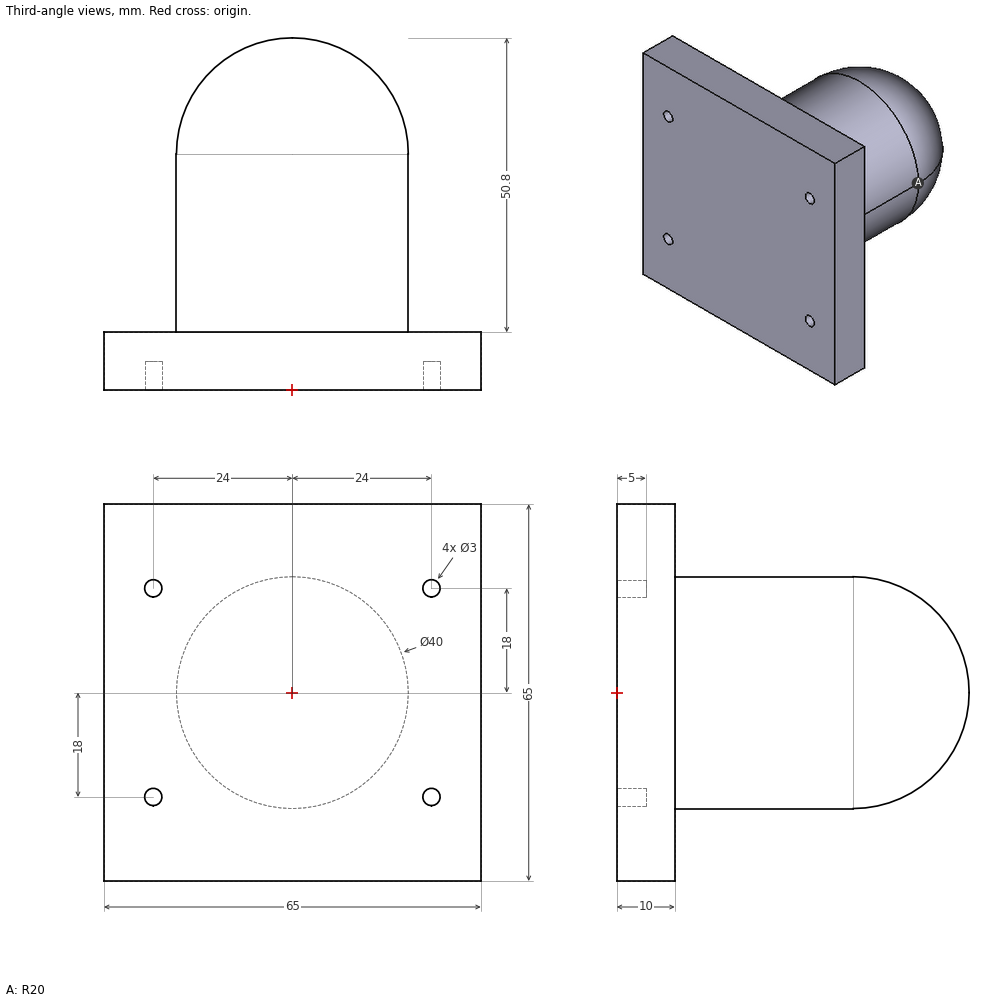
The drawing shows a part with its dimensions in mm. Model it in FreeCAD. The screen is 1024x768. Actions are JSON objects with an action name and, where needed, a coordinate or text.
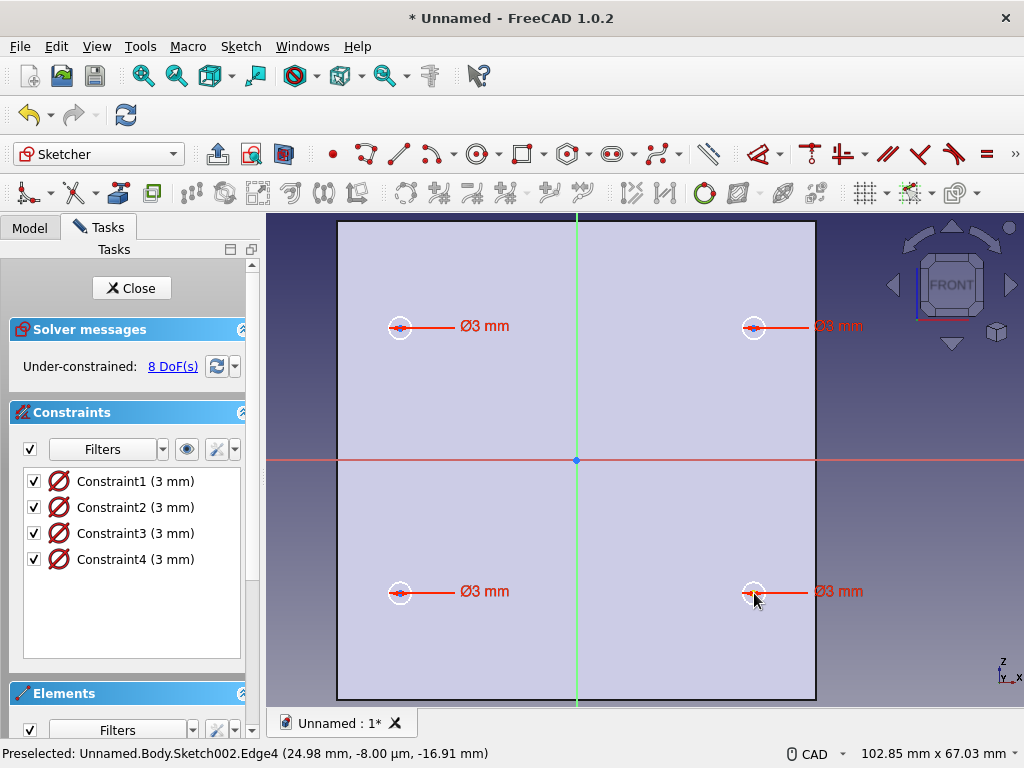
{"action": "left_click", "coordinate": [754, 328]}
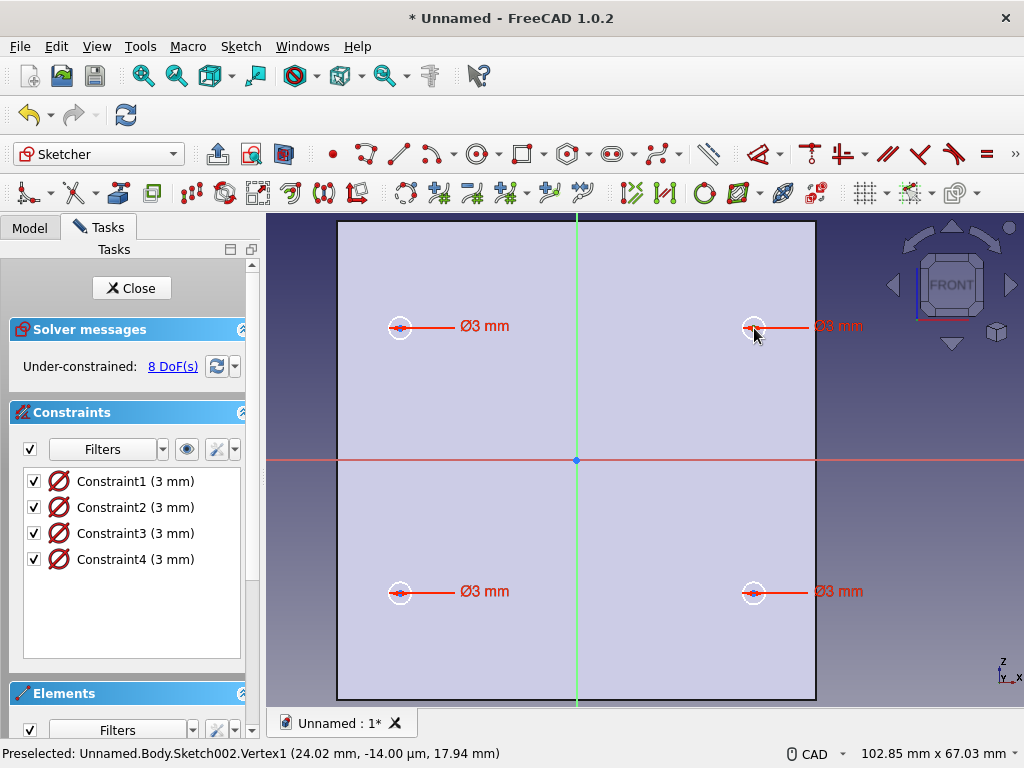
{"action": "left_click", "coordinate": [400, 328]}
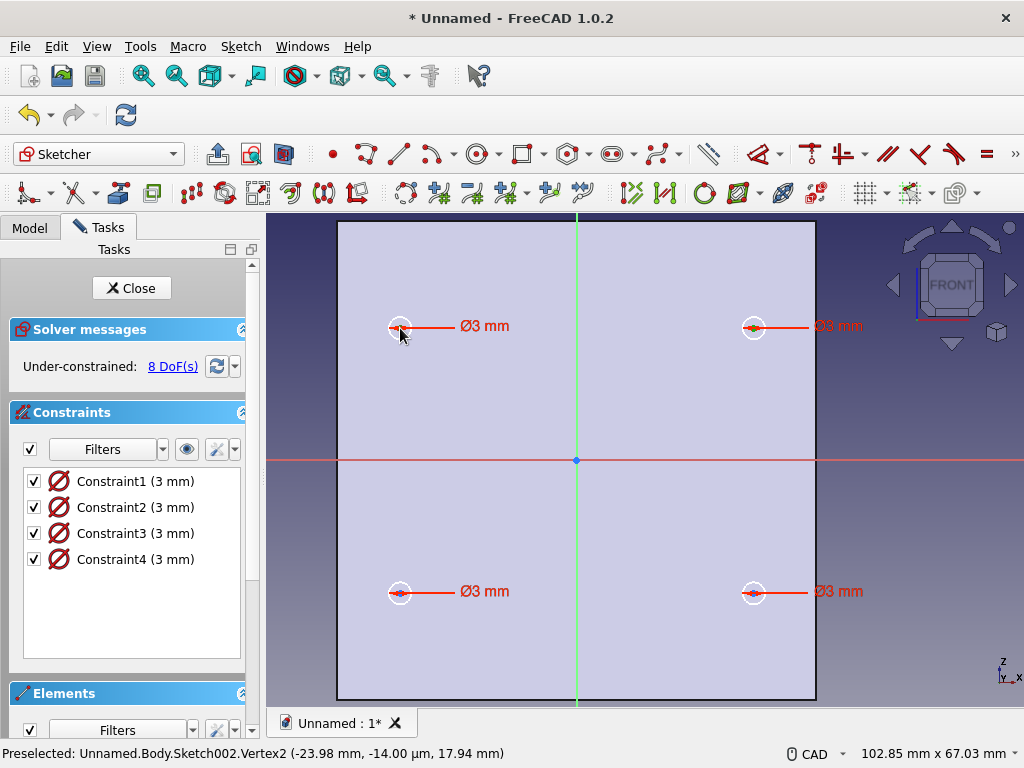
{"action": "key", "text": "h"}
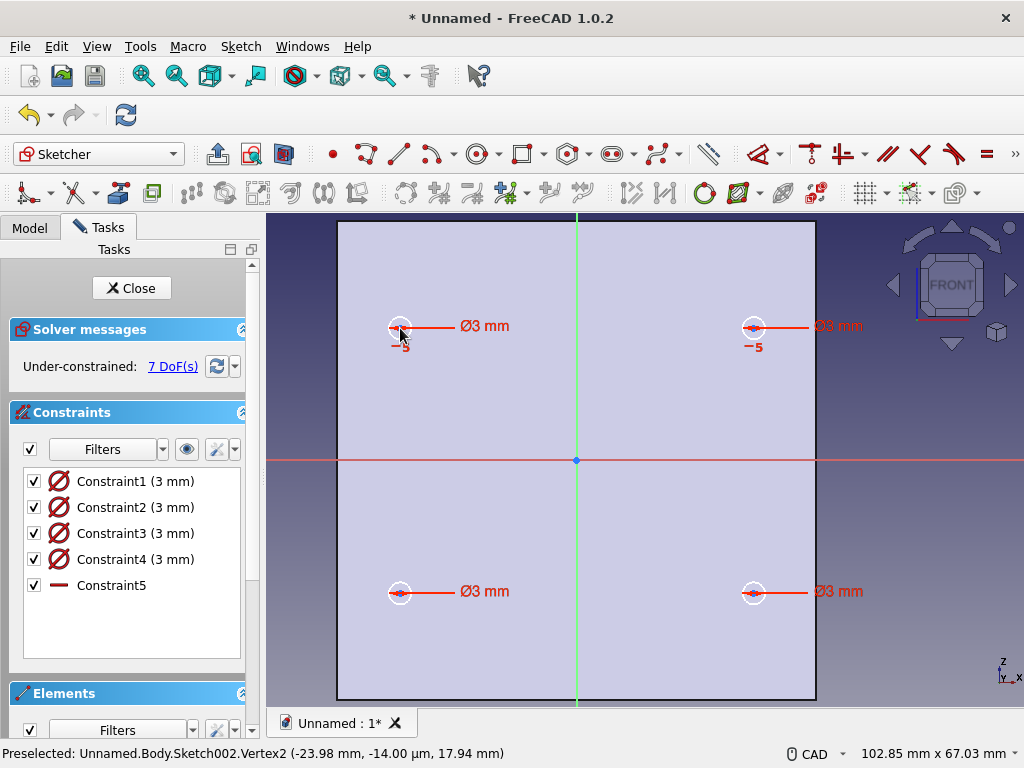
{"action": "left_click", "coordinate": [400, 328]}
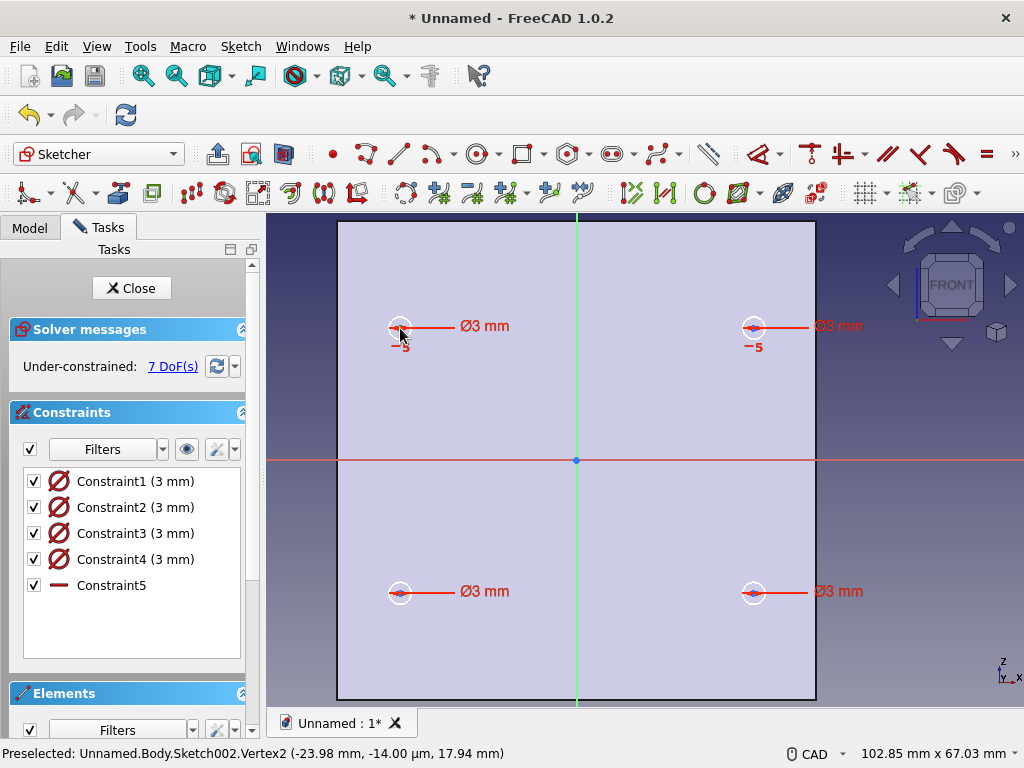
{"action": "left_click", "coordinate": [400, 593]}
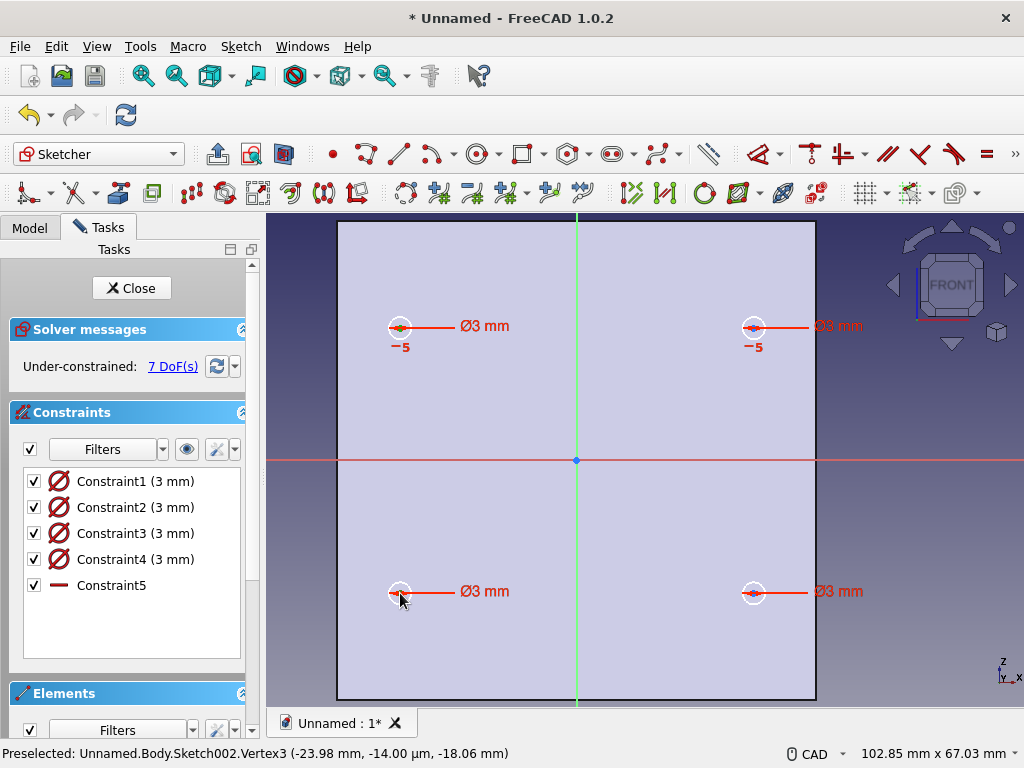
{"action": "left_click", "coordinate": [864, 154]}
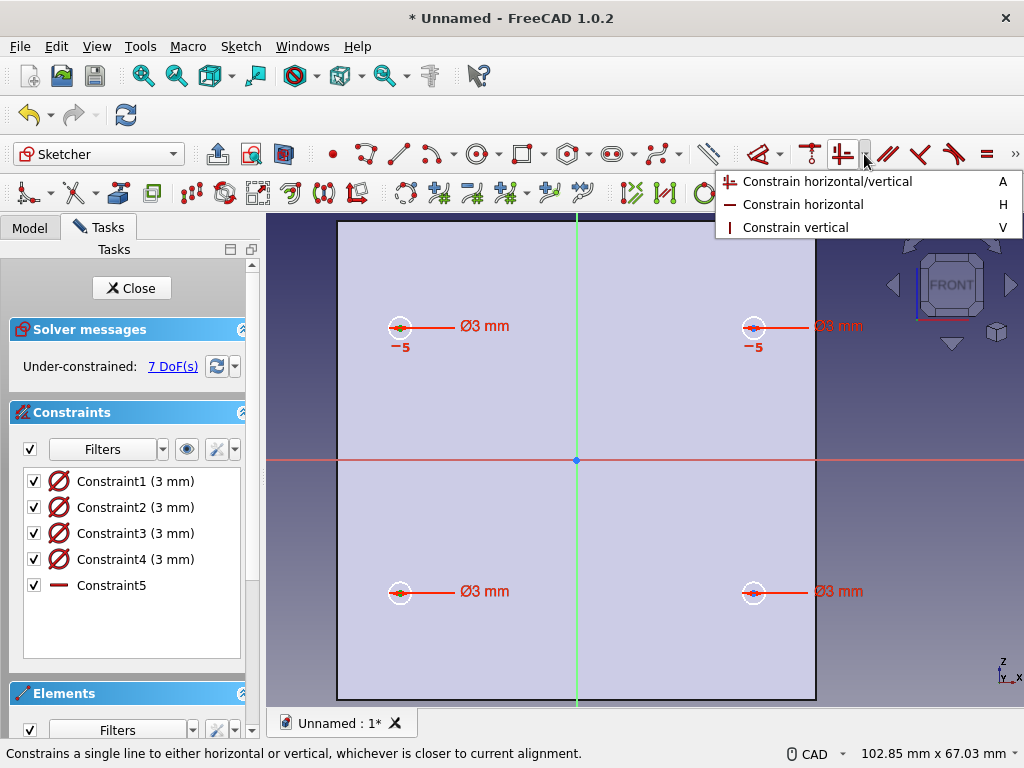
{"action": "left_click", "coordinate": [869, 228]}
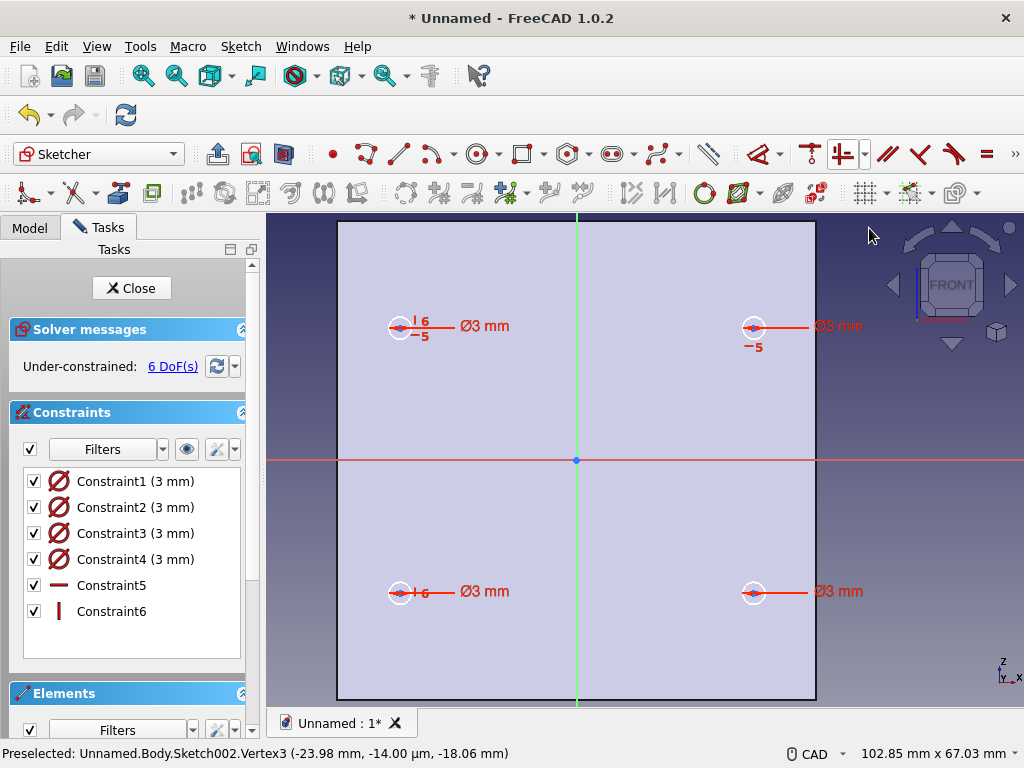
{"action": "left_click", "coordinate": [754, 328]}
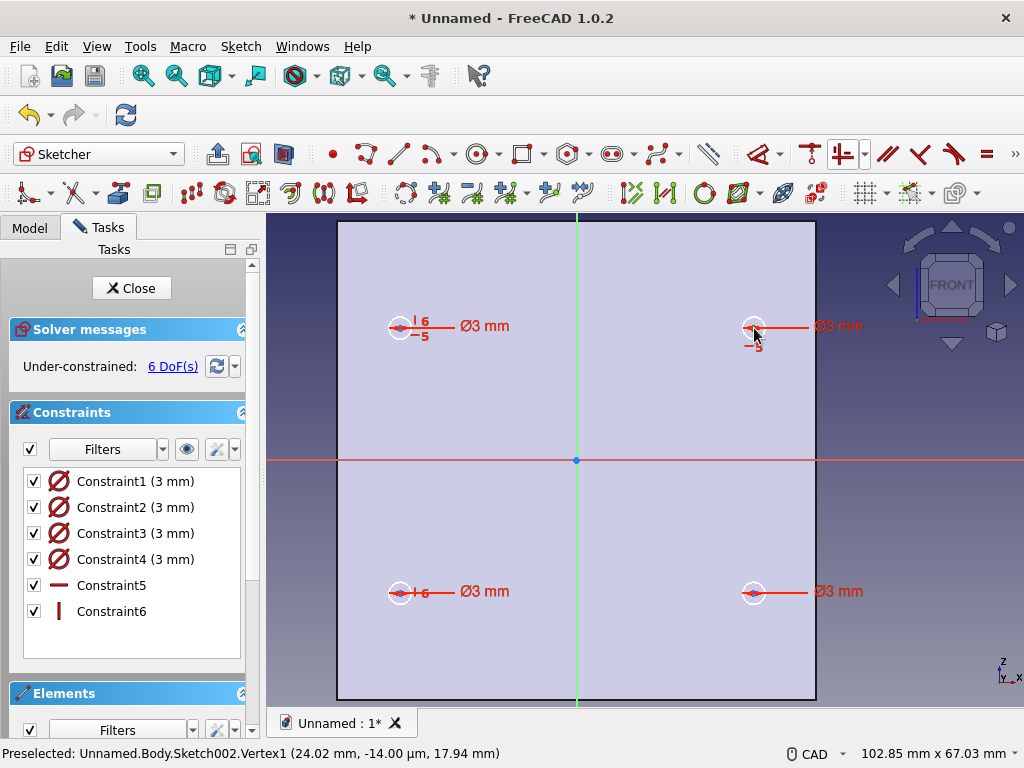
{"action": "left_click", "coordinate": [754, 593]}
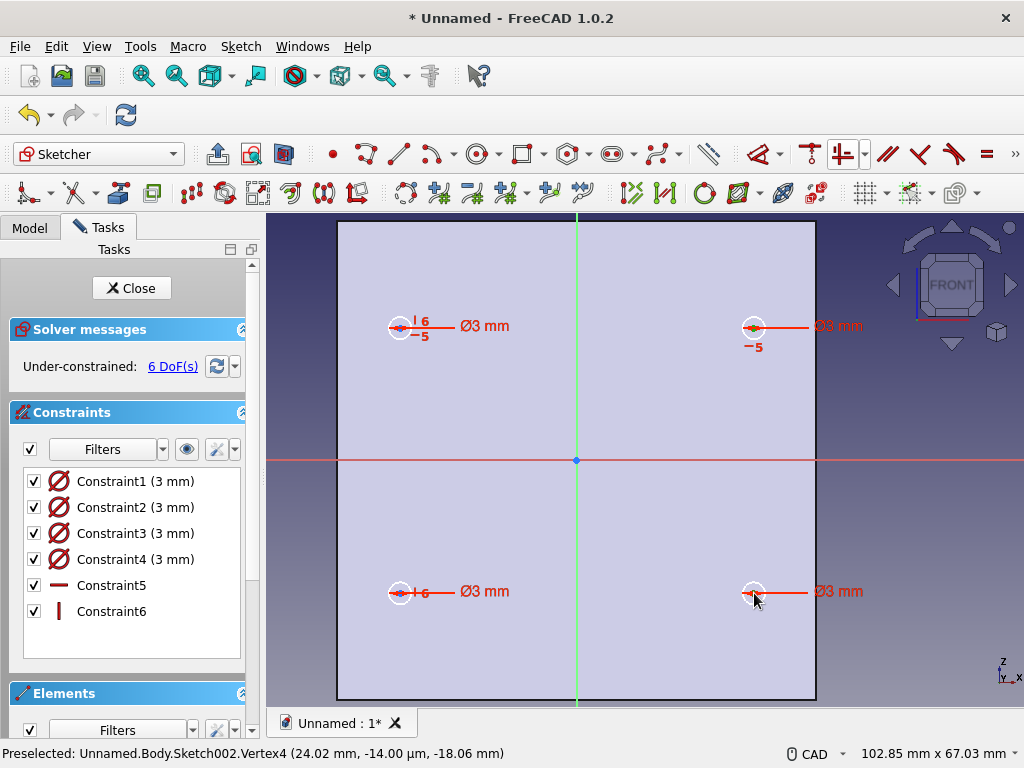
{"action": "key", "text": "v"}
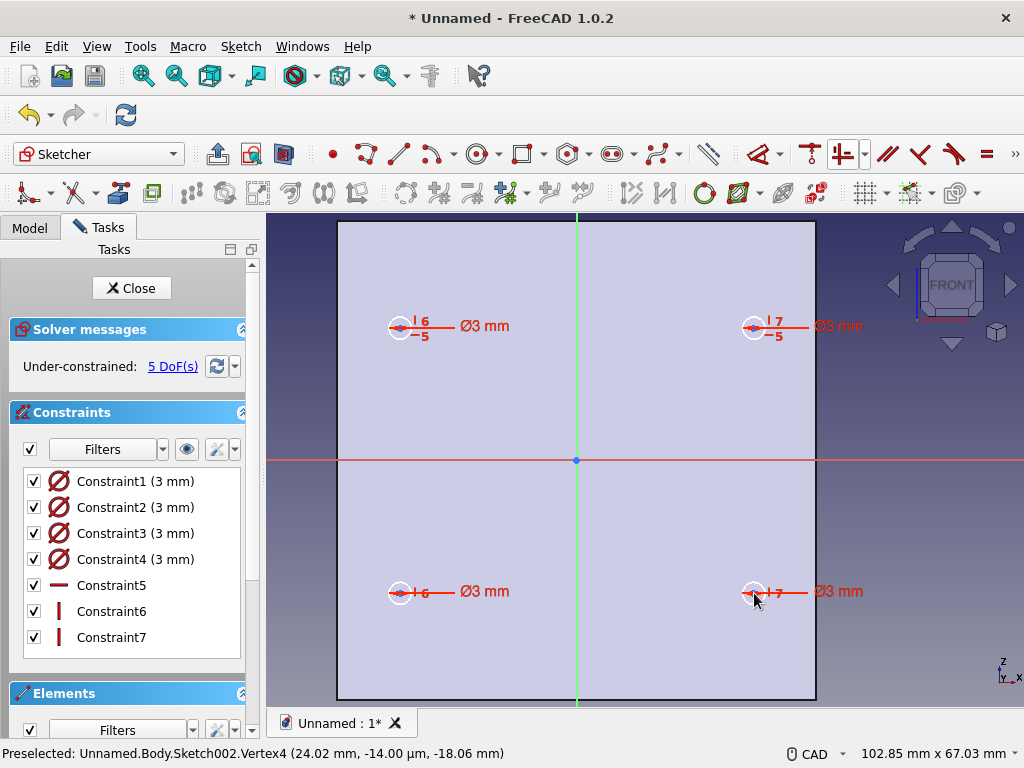
{"action": "left_click", "coordinate": [400, 593]}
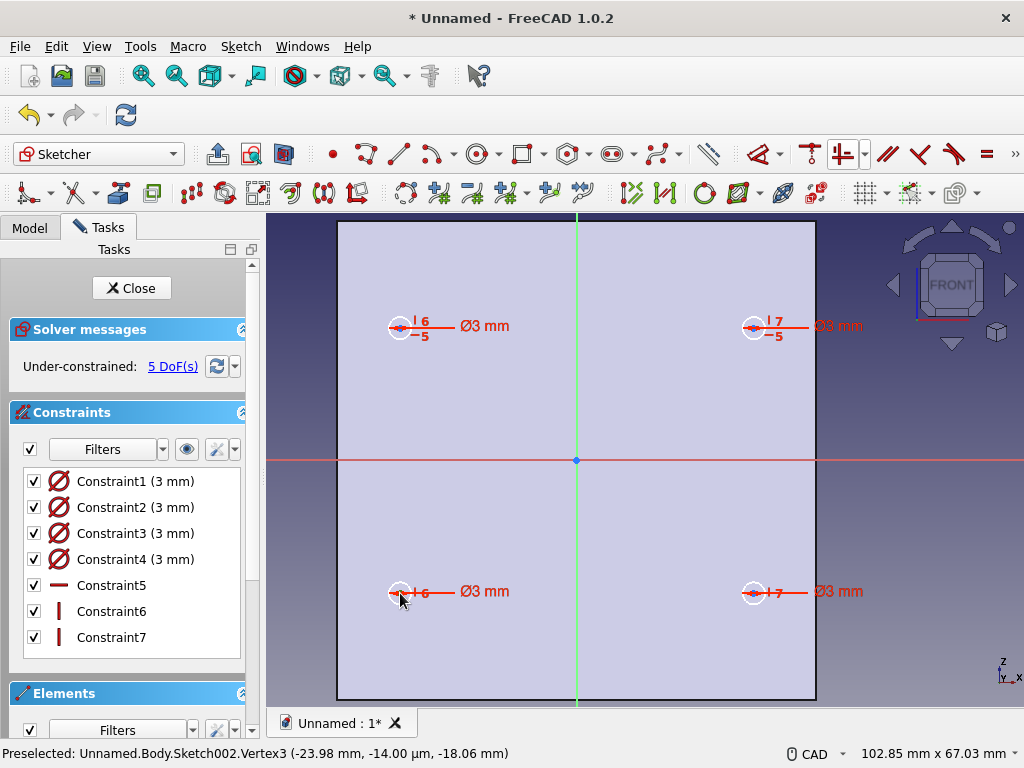
{"action": "left_click", "coordinate": [754, 593]}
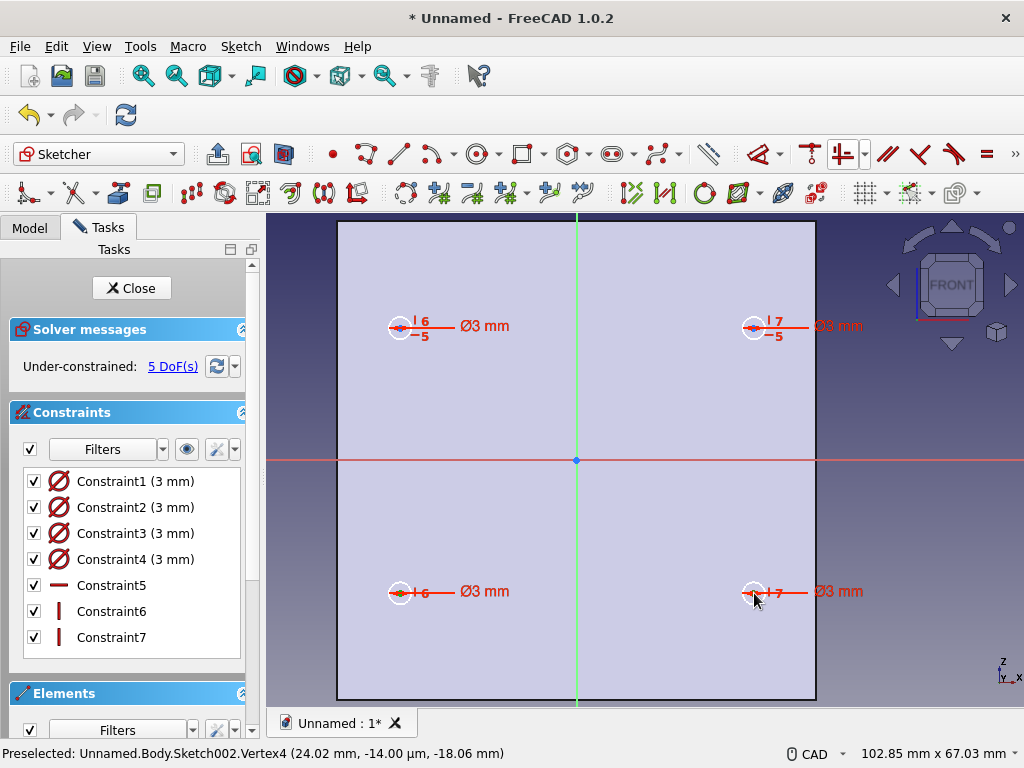
{"action": "key", "text": "h"}